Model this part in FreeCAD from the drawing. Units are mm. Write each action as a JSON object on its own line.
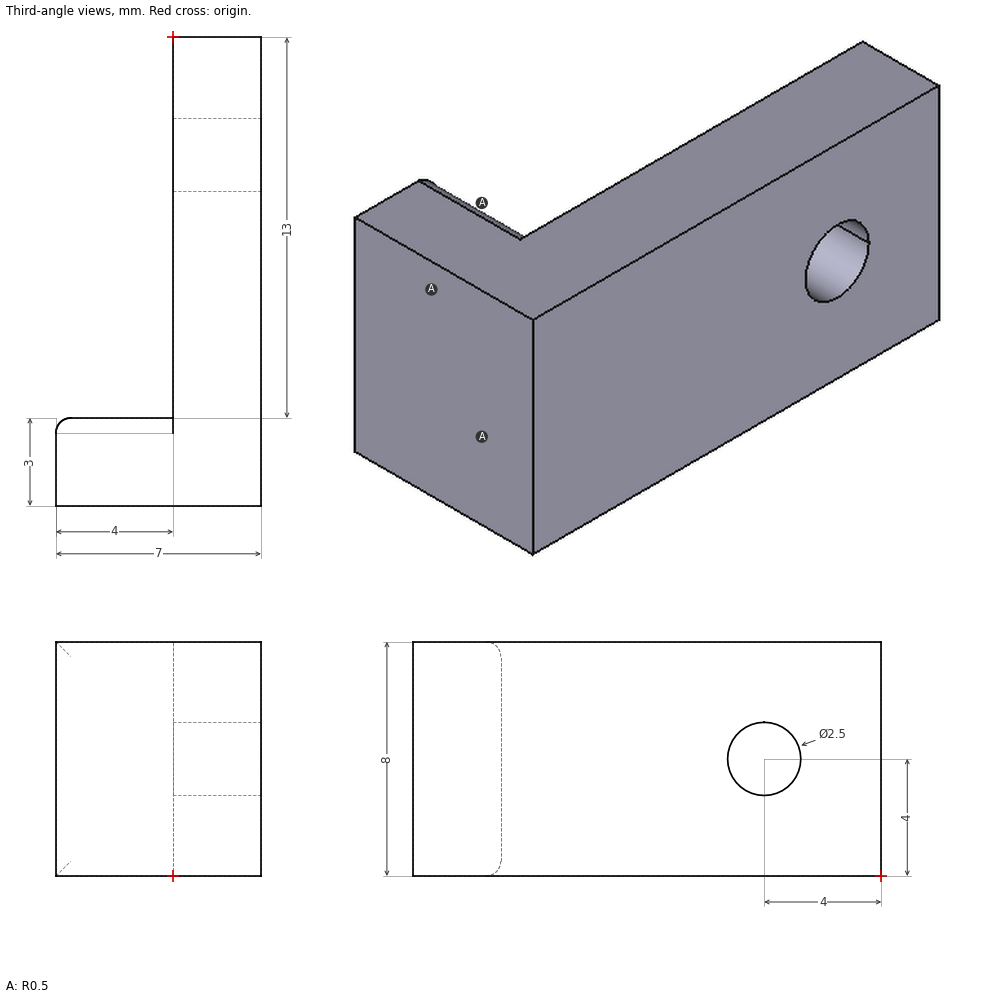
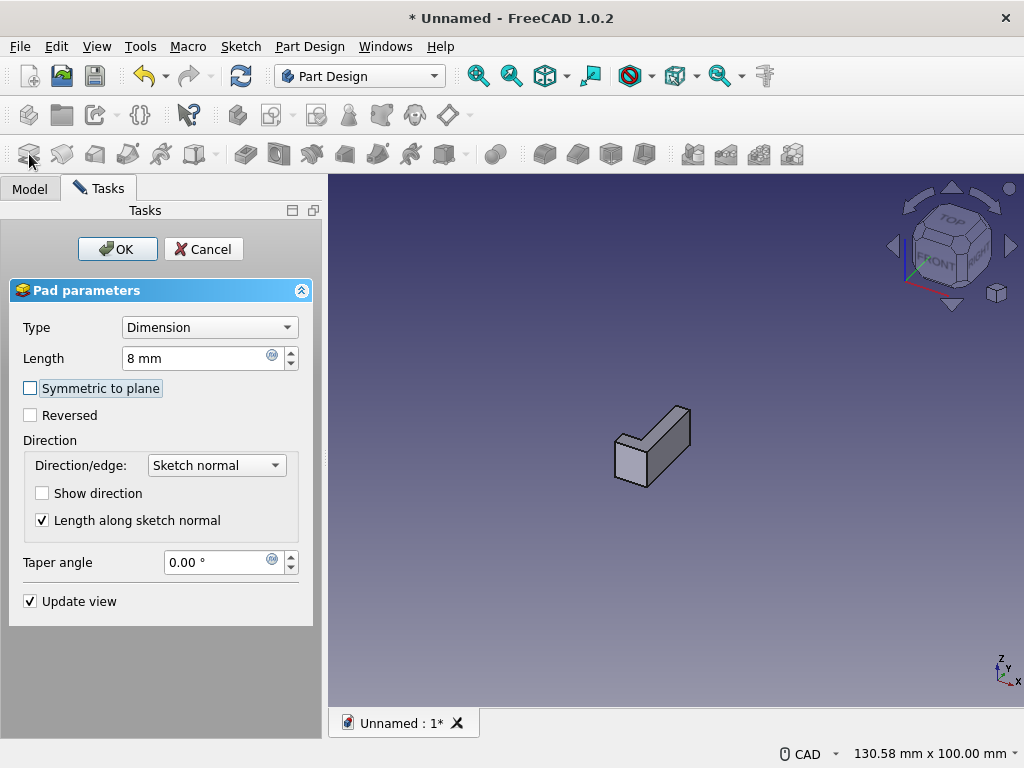
{"action": "left_click", "coordinate": [118, 249]}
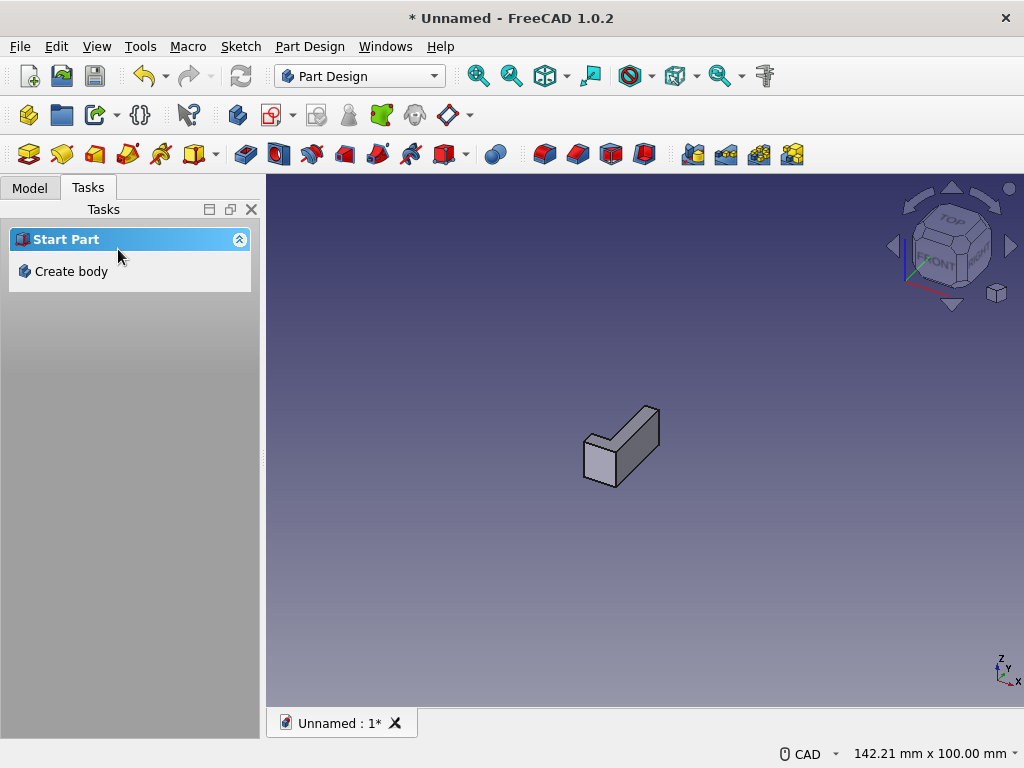
{"action": "left_click", "coordinate": [479, 76]}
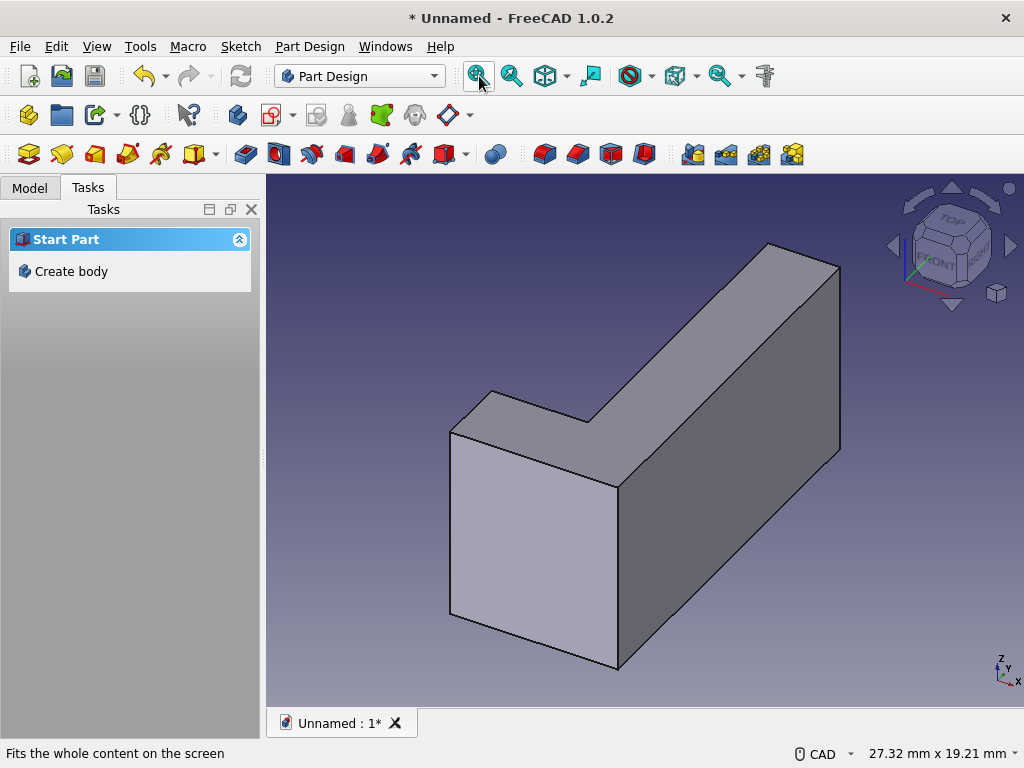
{"action": "left_click", "coordinate": [761, 436]}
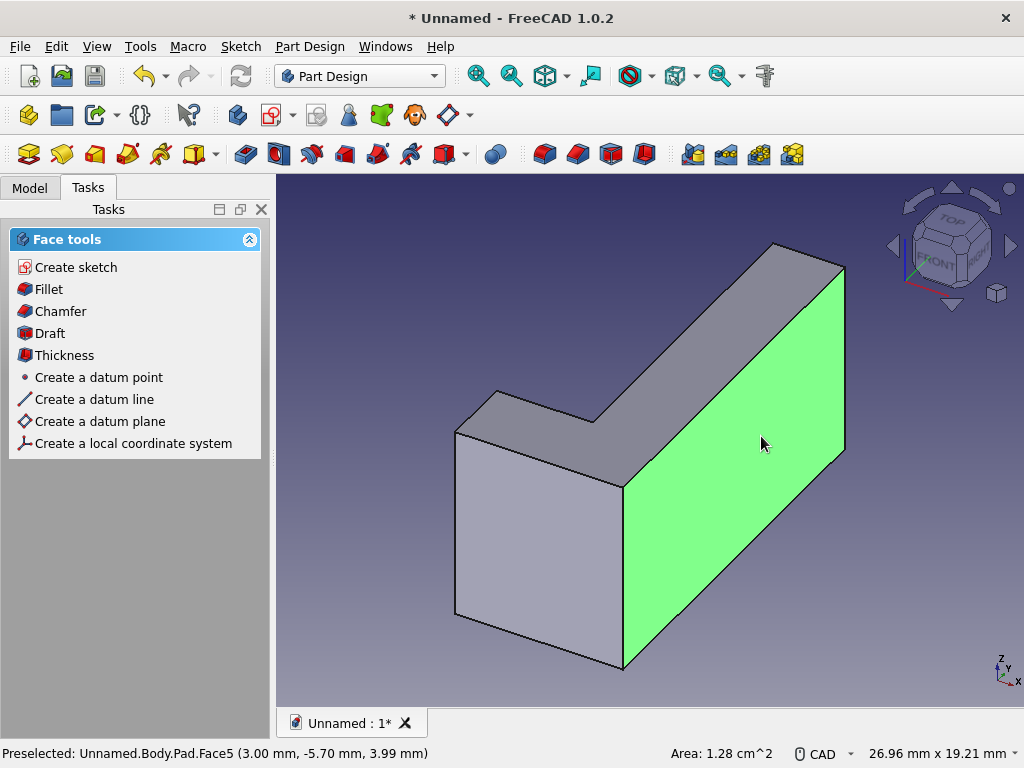
{"action": "left_click", "coordinate": [270, 116]}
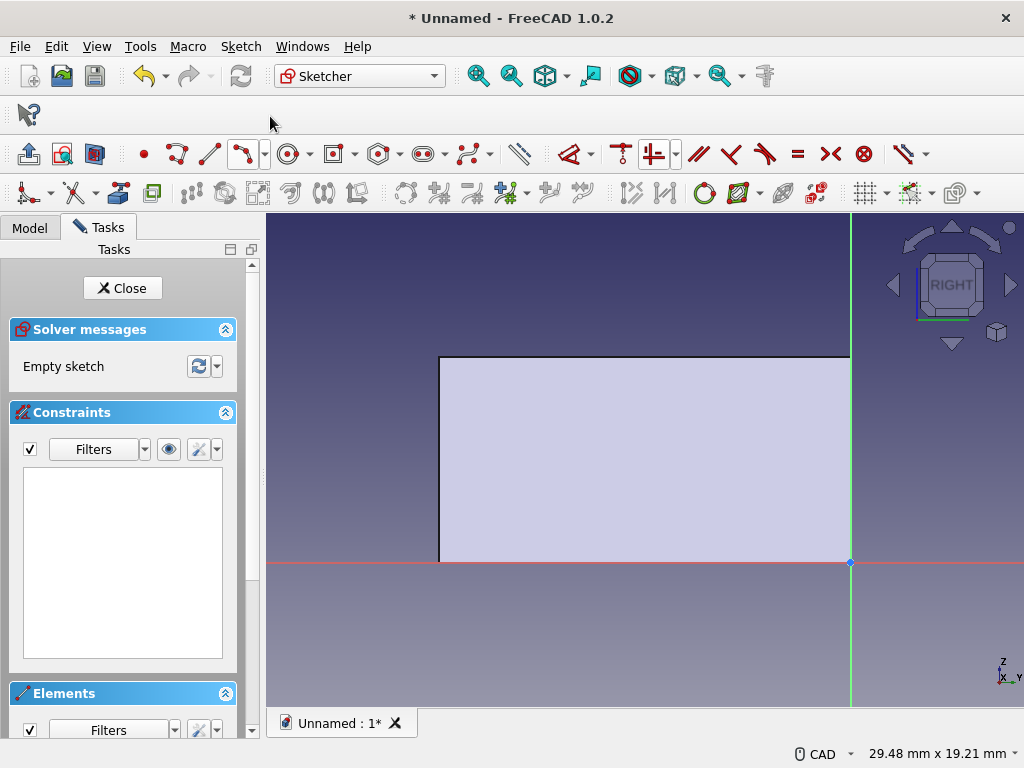
{"action": "scroll", "coordinate": [576, 460], "scroll_direction": "down", "scroll_amount": 5}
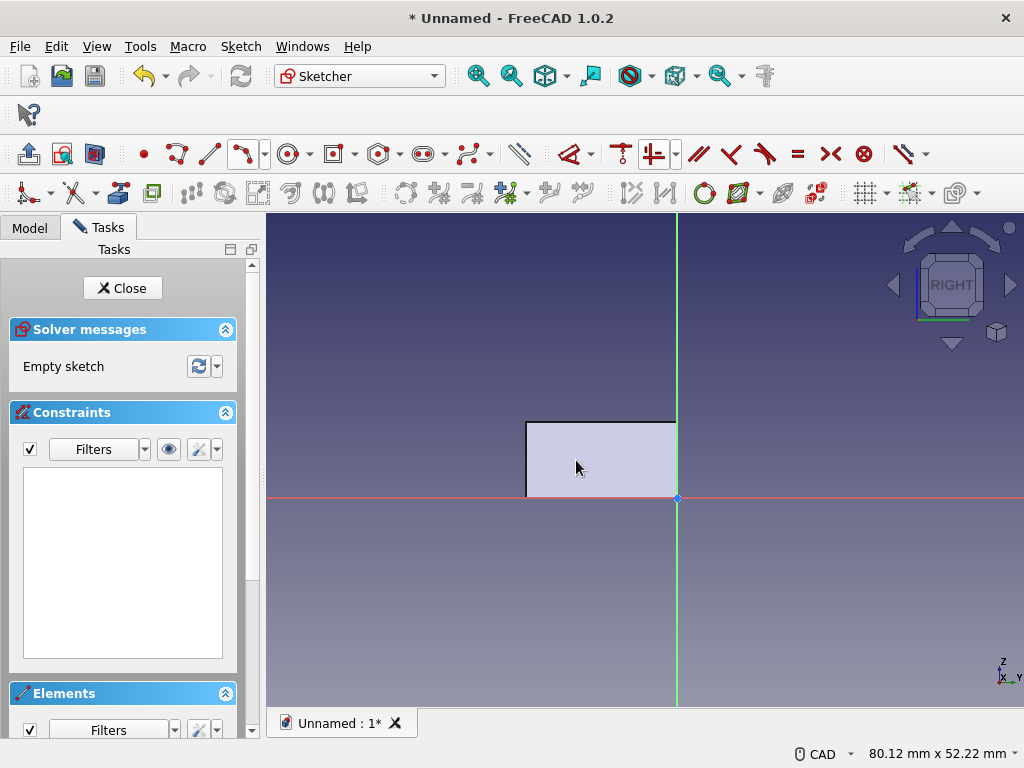
{"action": "scroll", "coordinate": [668, 476], "scroll_direction": "up", "scroll_amount": 9}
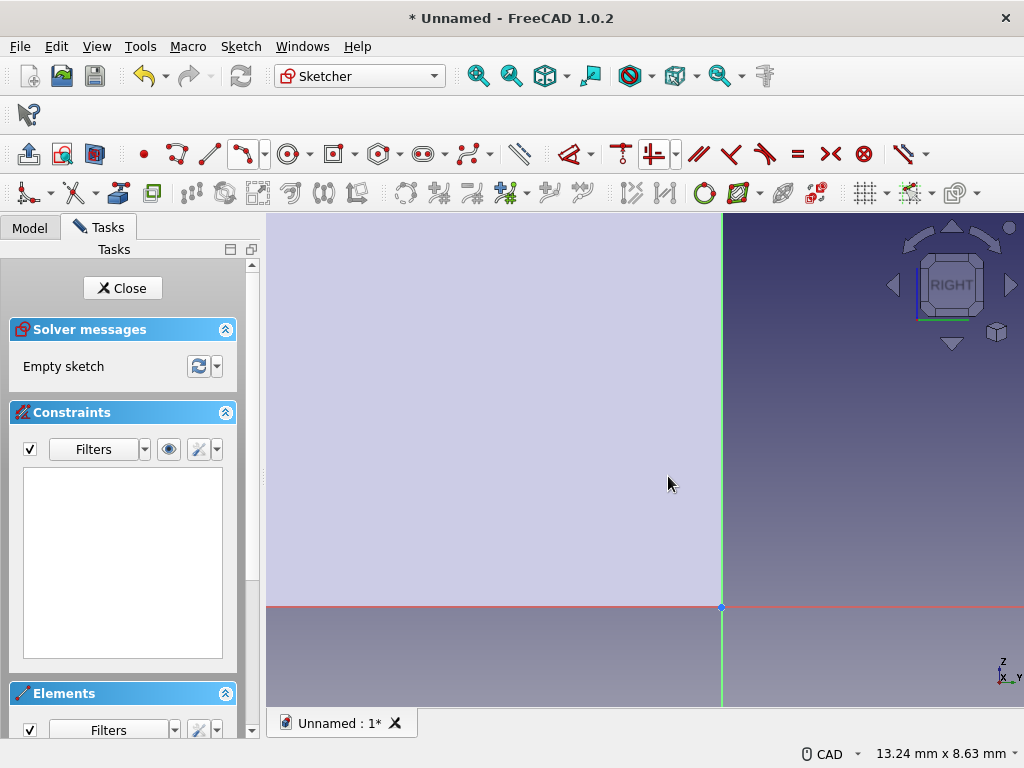
{"action": "left_click", "coordinate": [288, 154]}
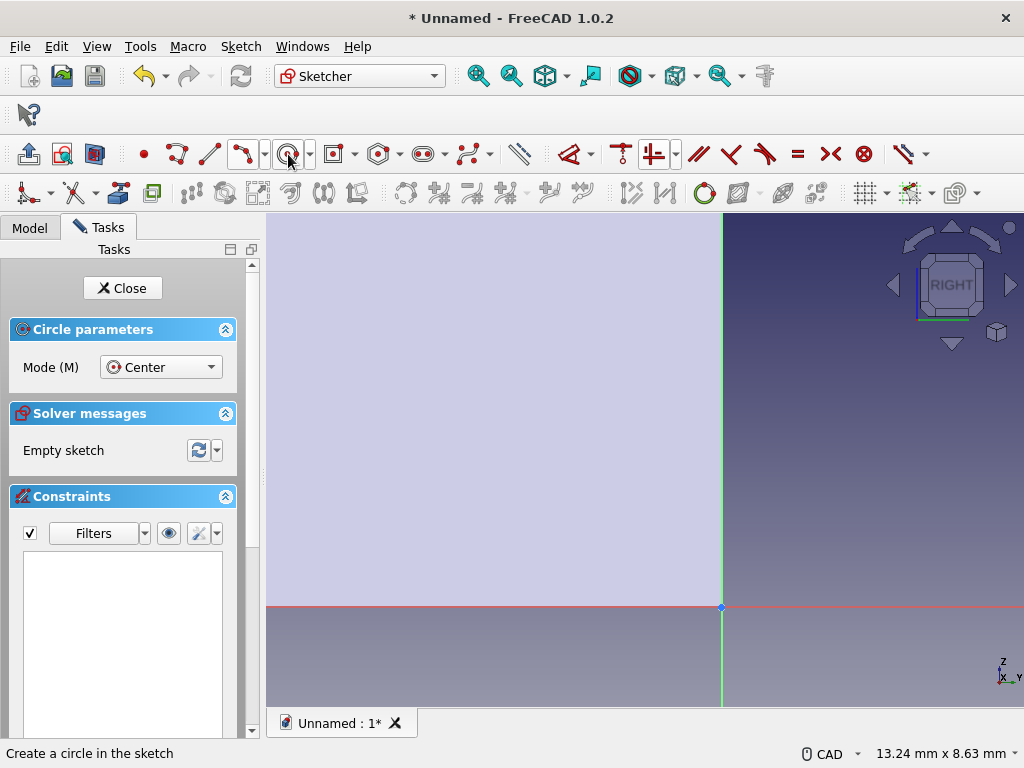
{"action": "left_click", "coordinate": [493, 378]}
{"action": "left_click", "coordinate": [543, 328]}
{"action": "key", "text": "Escape"}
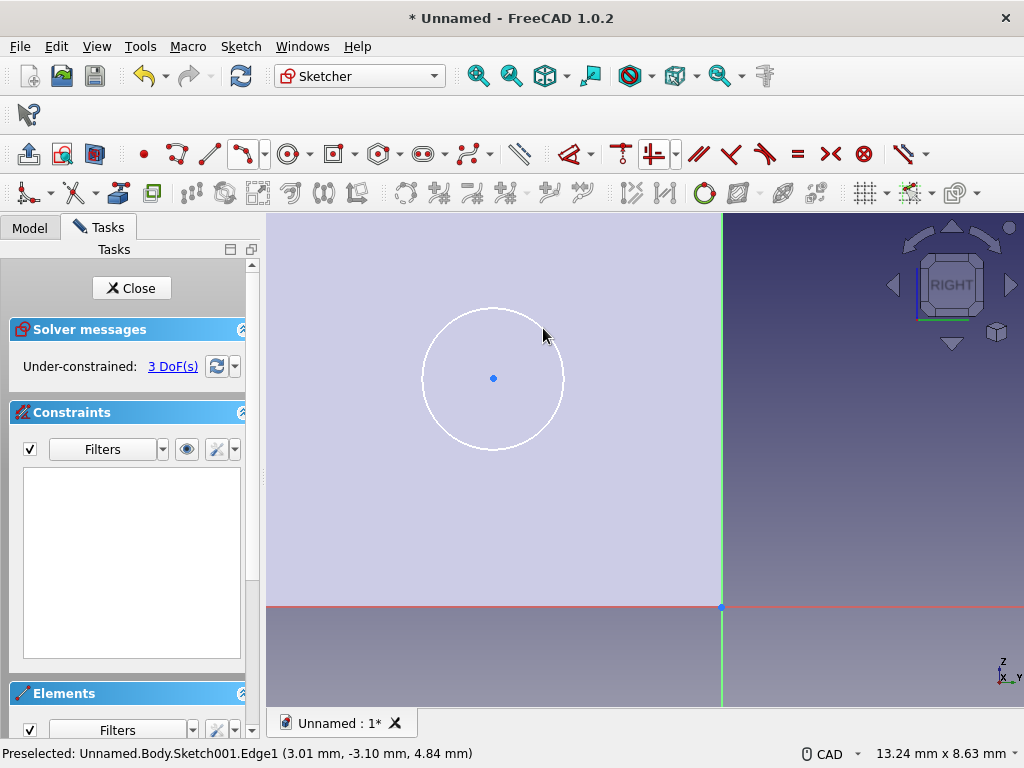
{"action": "key", "text": "d"}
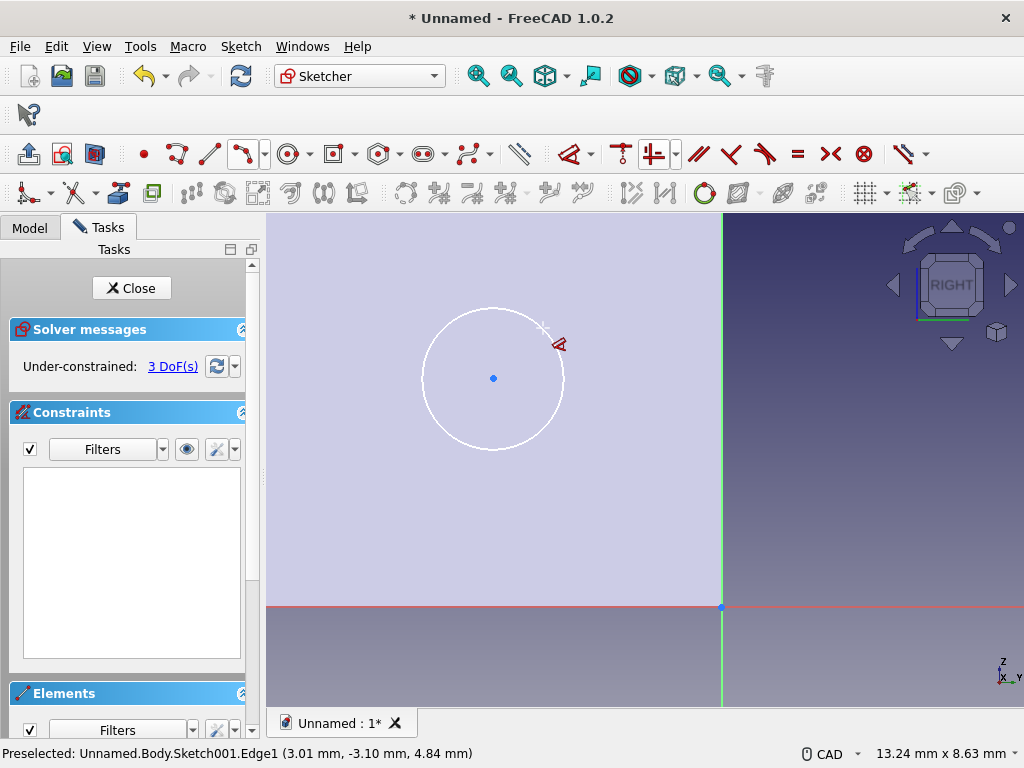
{"action": "left_click", "coordinate": [543, 329]}
{"action": "left_click", "coordinate": [566, 306]}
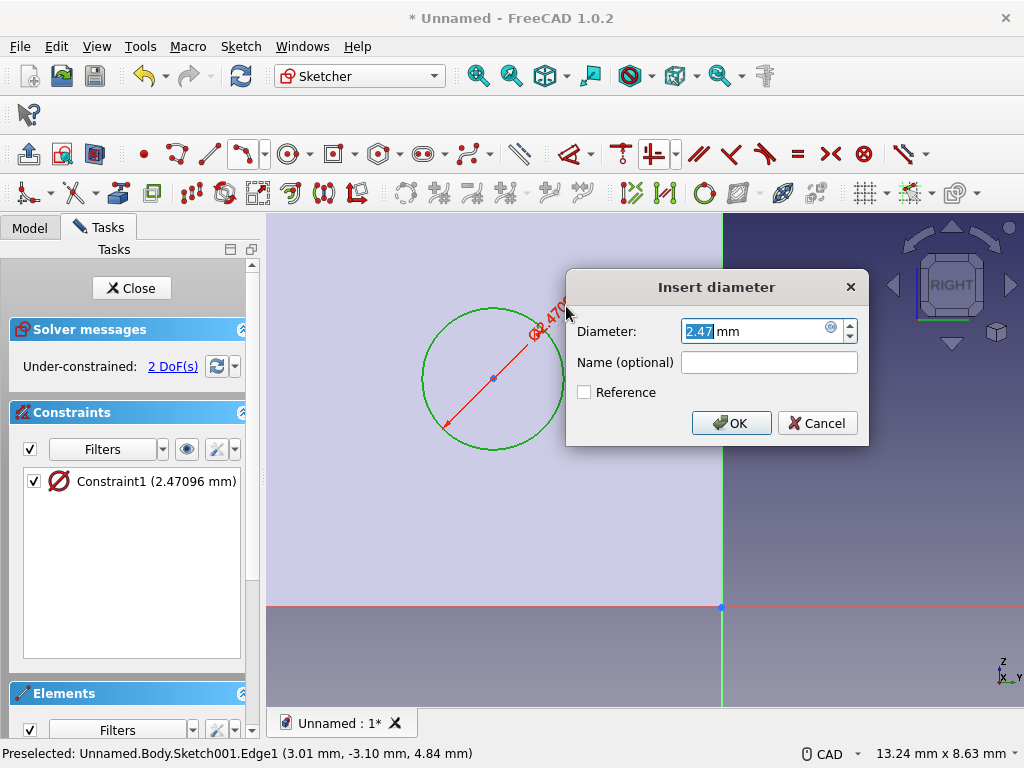
{"action": "type", "text": "2.5"}
{"action": "key", "text": "Return"}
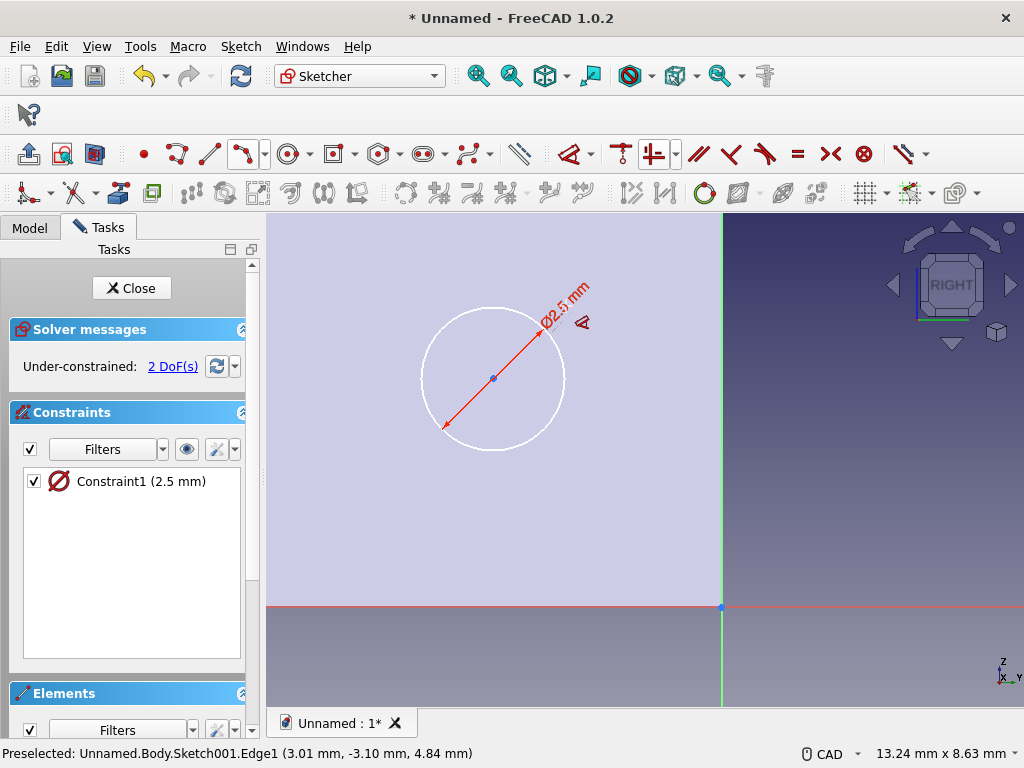
{"action": "left_click", "coordinate": [493, 379]}
{"action": "left_click", "coordinate": [607, 641]}